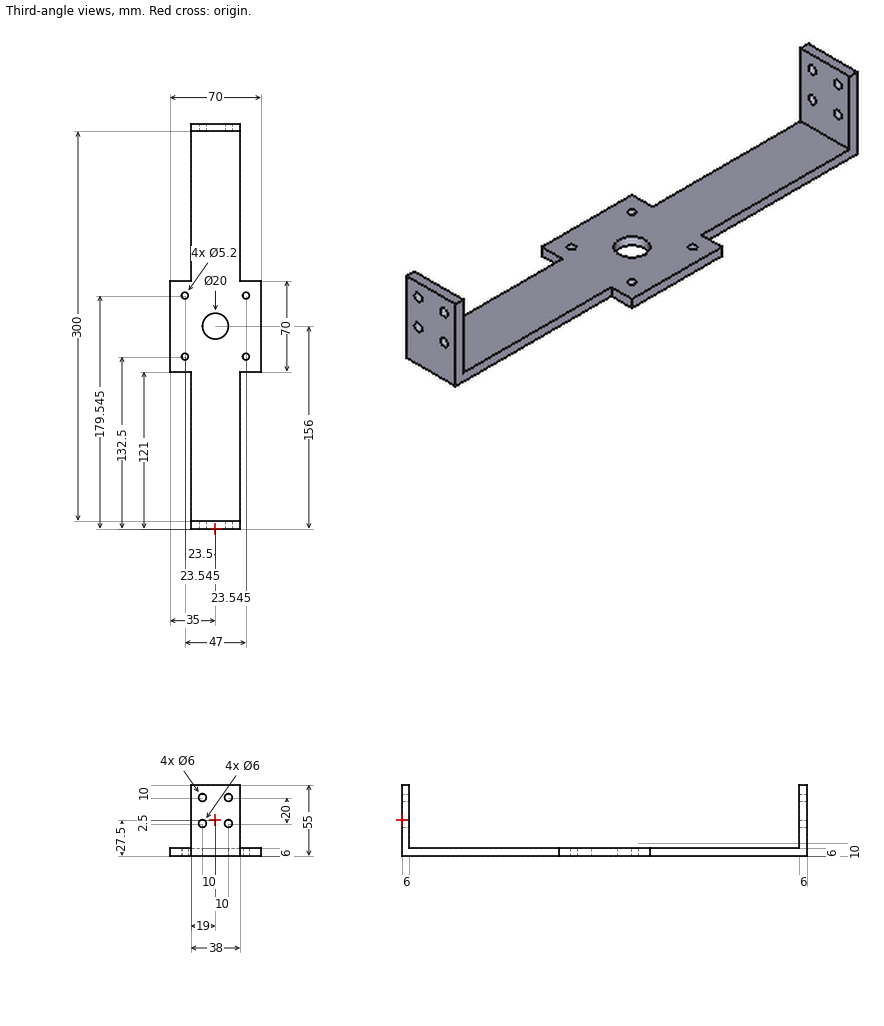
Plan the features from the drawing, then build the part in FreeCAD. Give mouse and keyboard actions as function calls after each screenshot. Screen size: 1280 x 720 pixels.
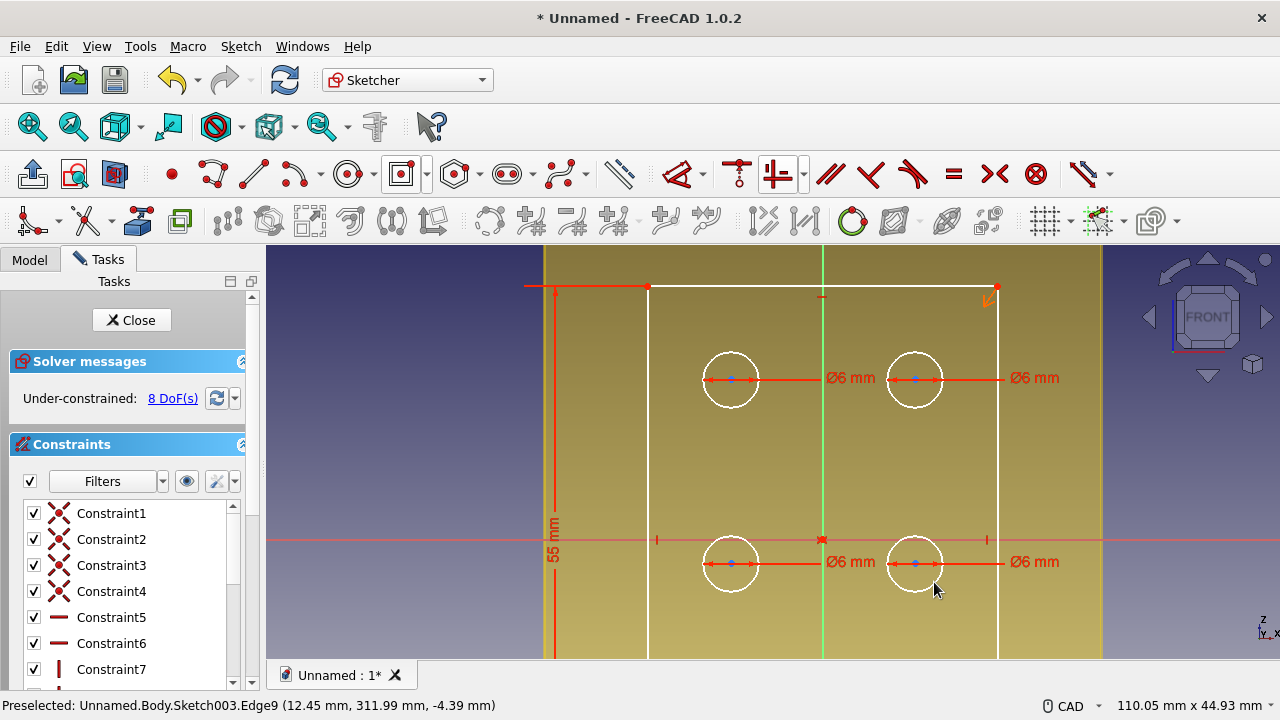
click(731, 380)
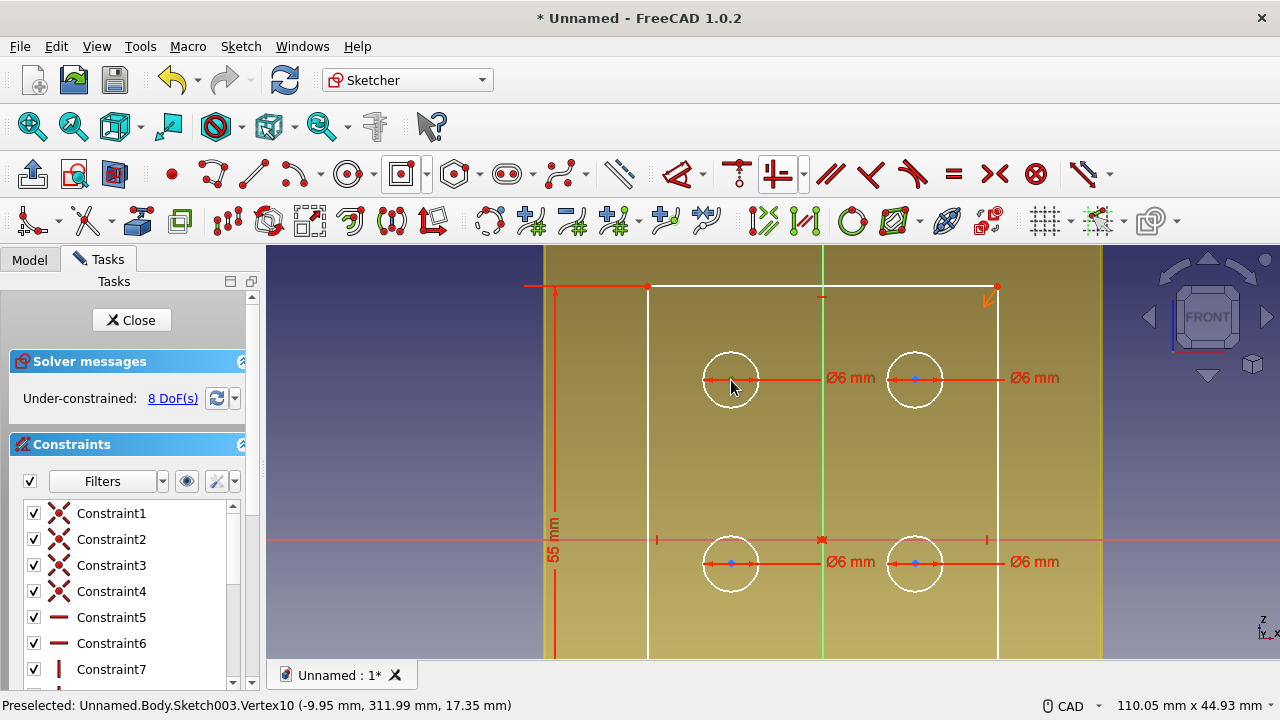
click(915, 380)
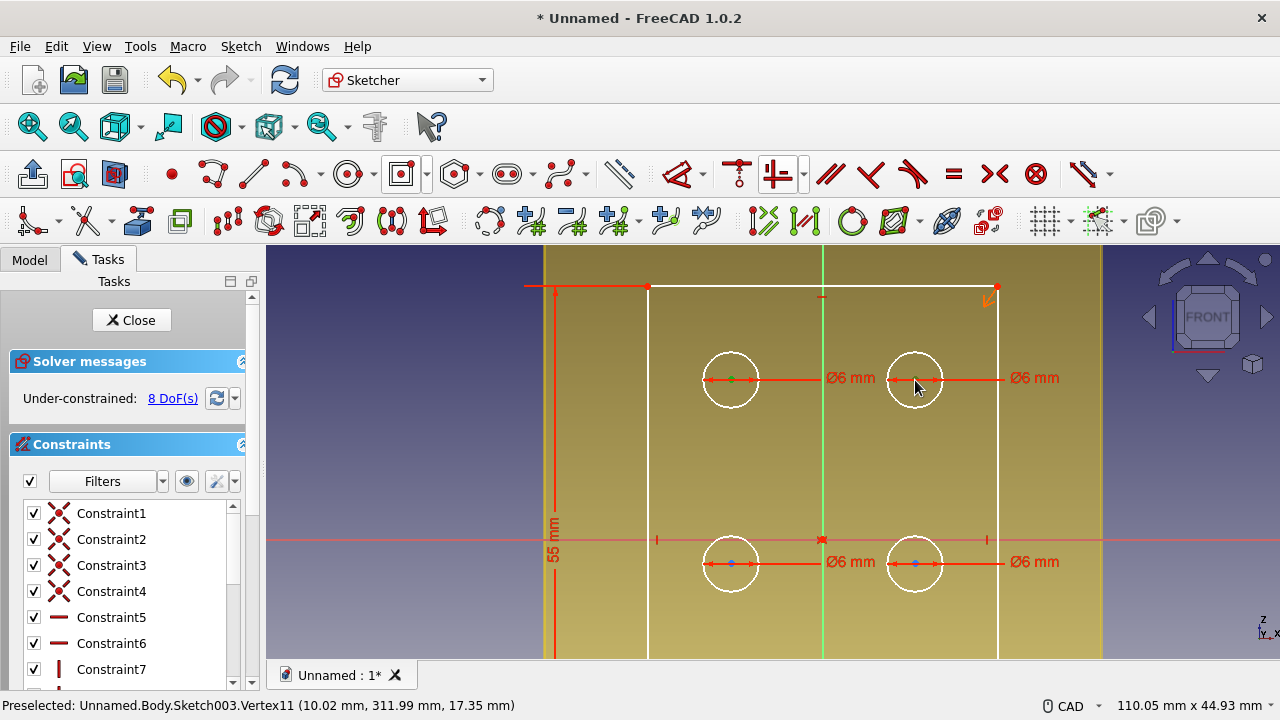
click(804, 174)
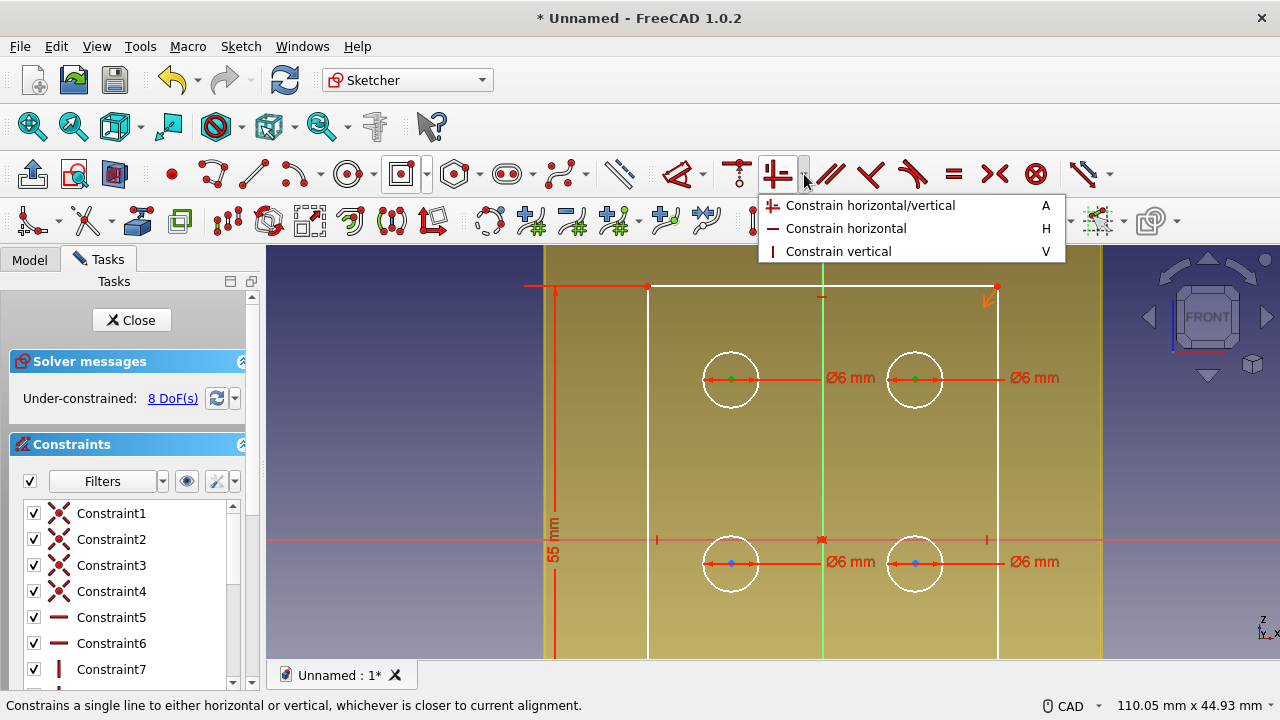
click(912, 228)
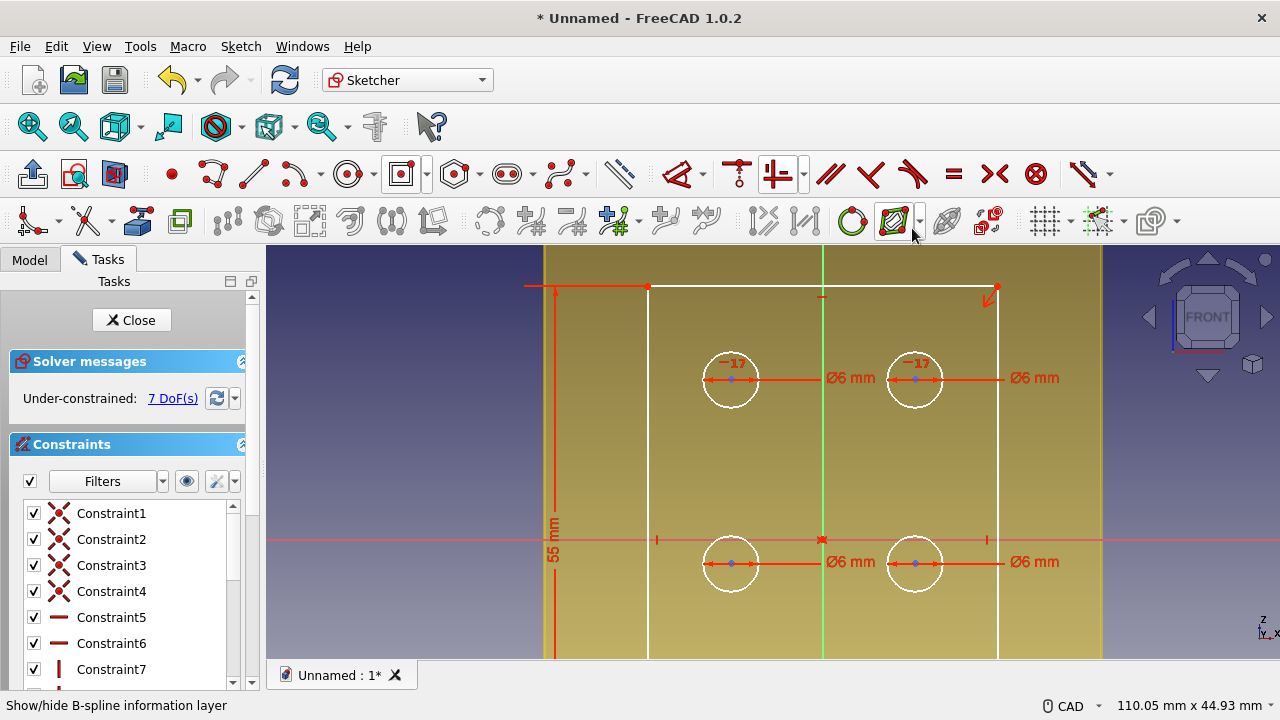
click(731, 380)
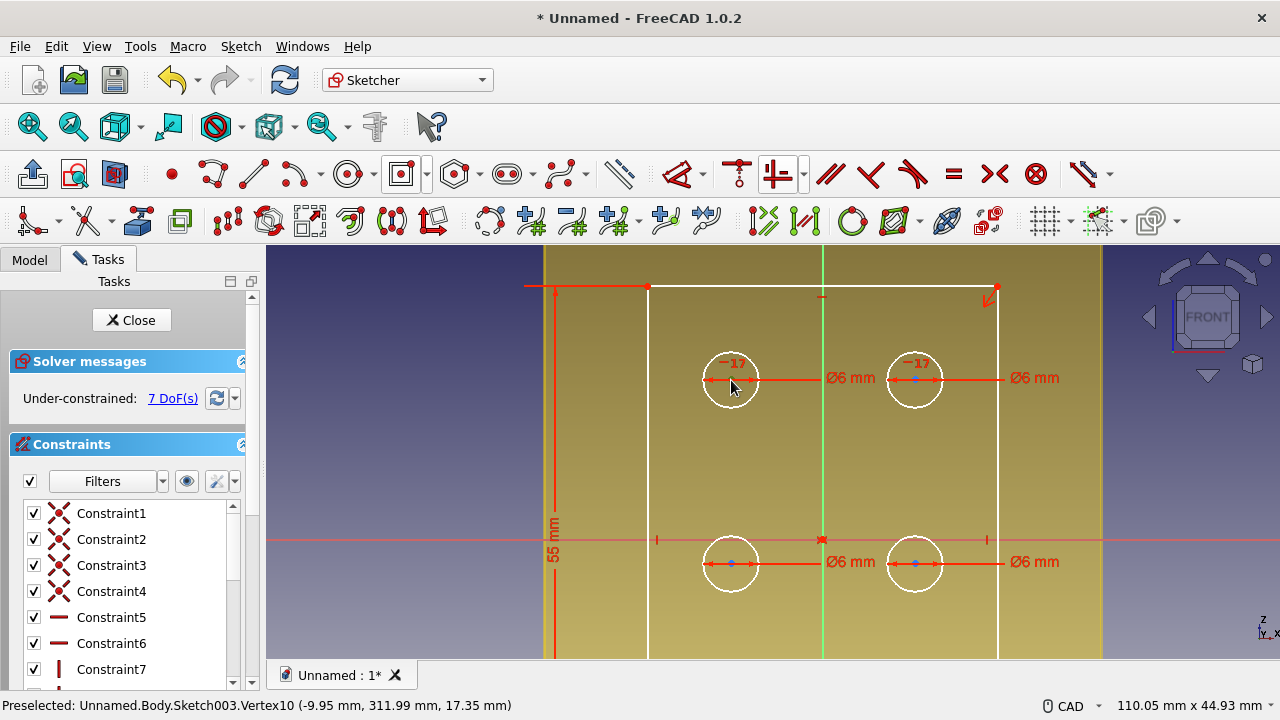
click(731, 564)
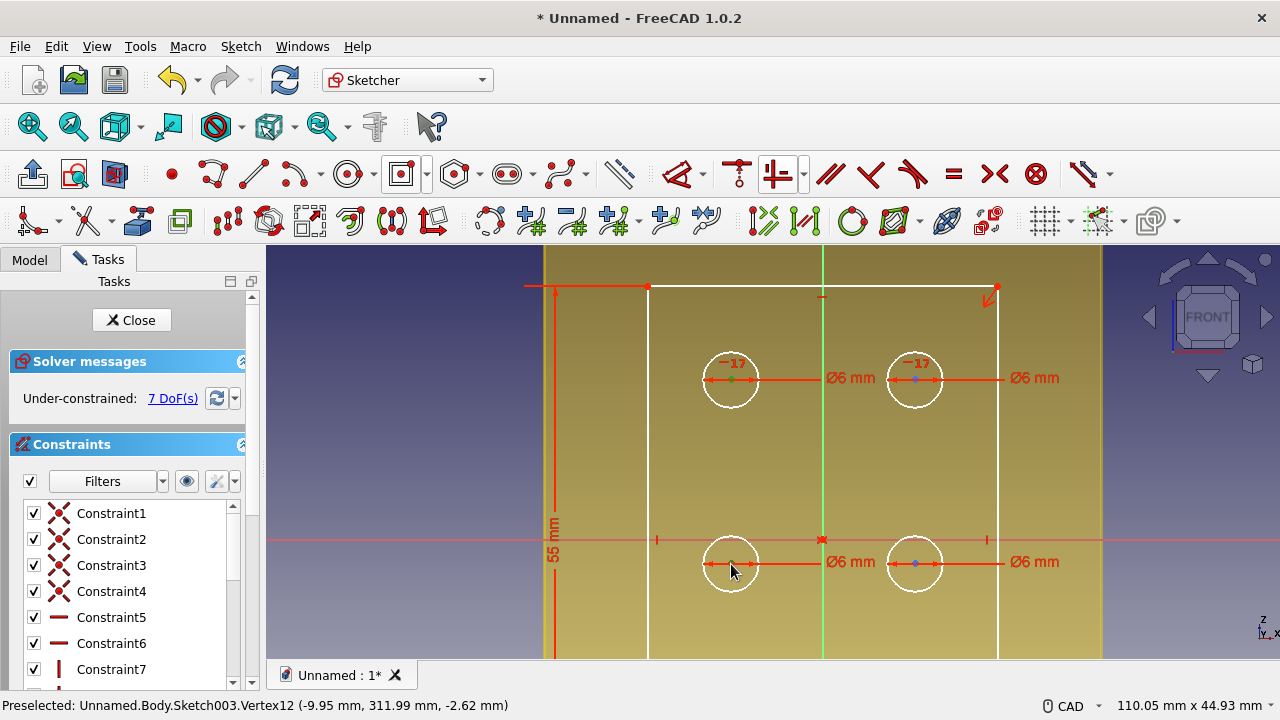
click(804, 174)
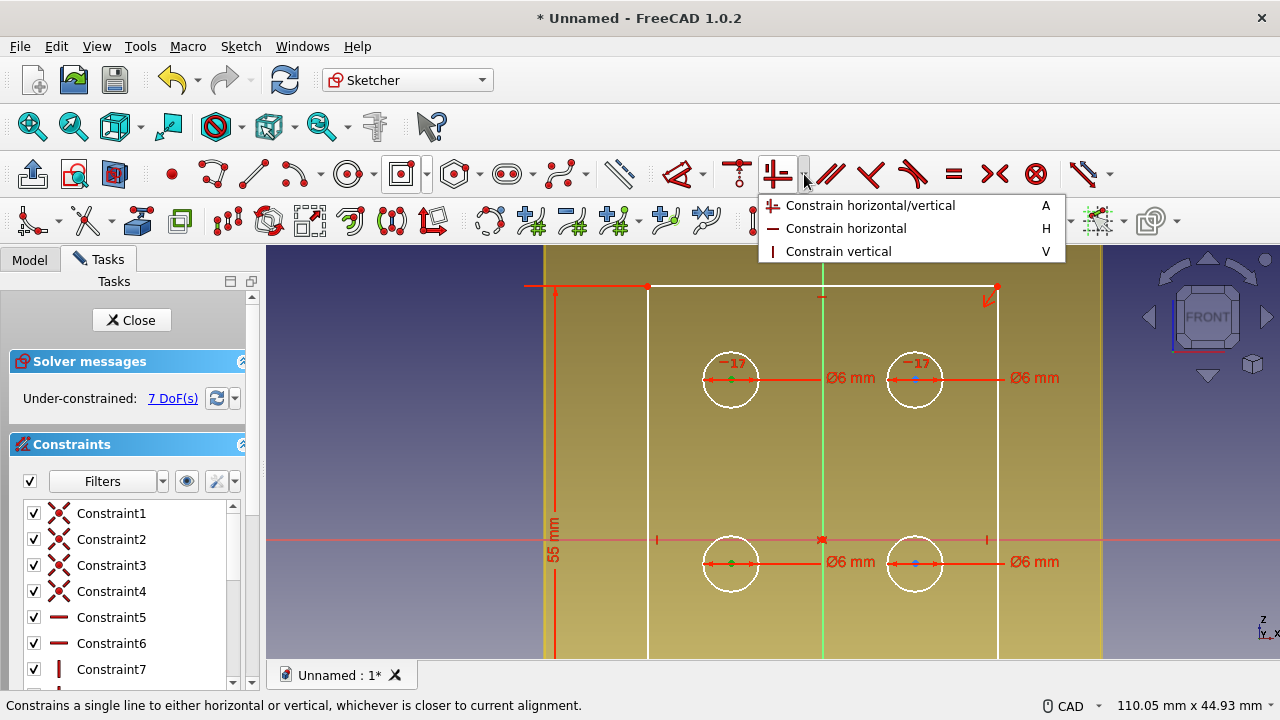
click(912, 252)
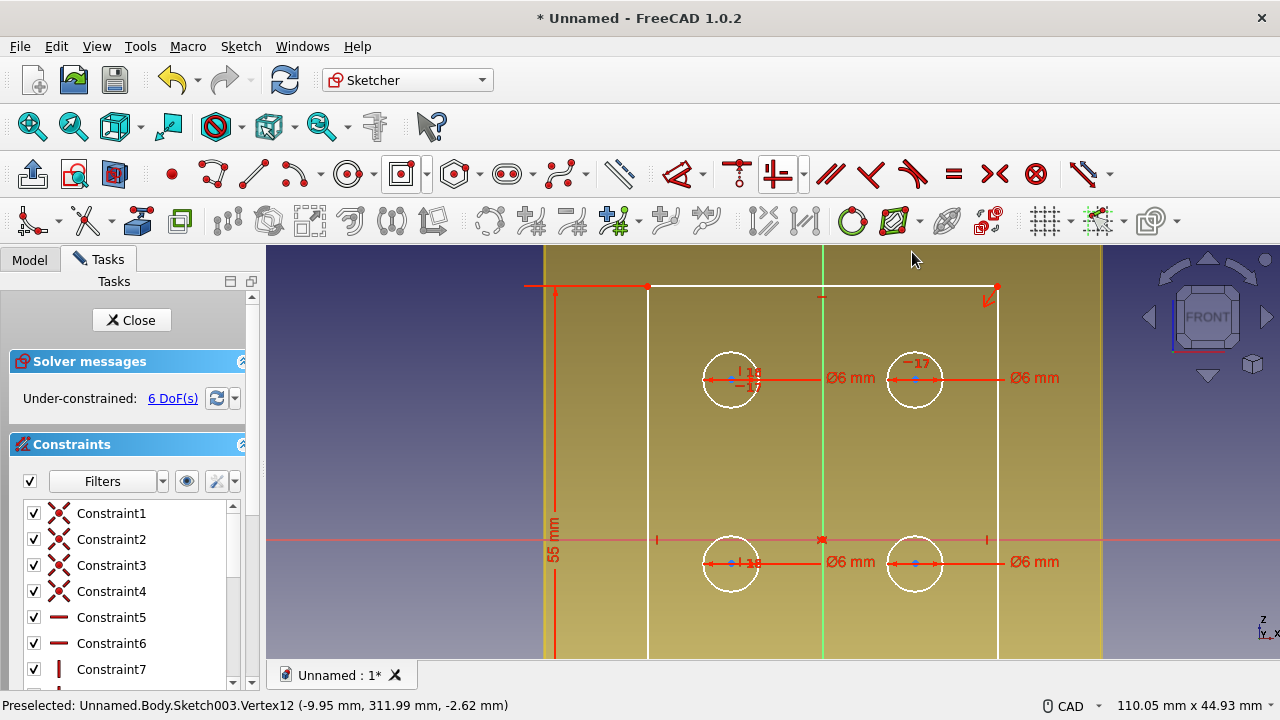
click(915, 380)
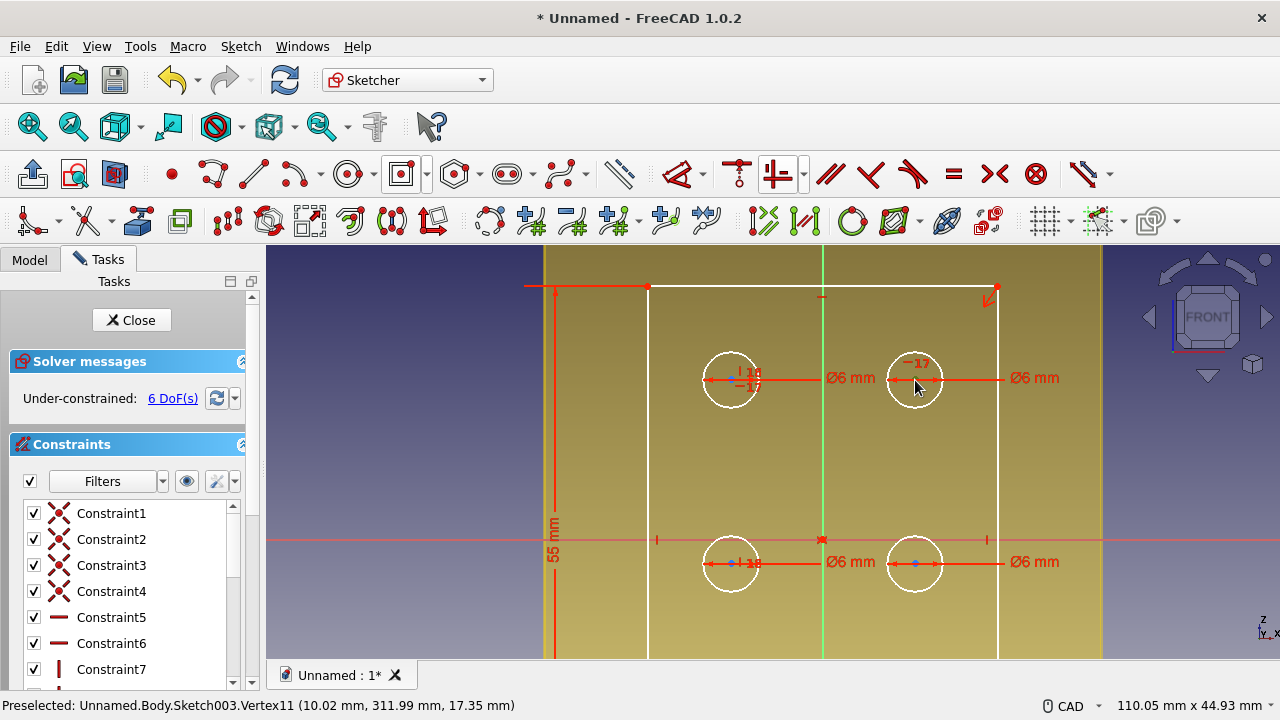
click(915, 564)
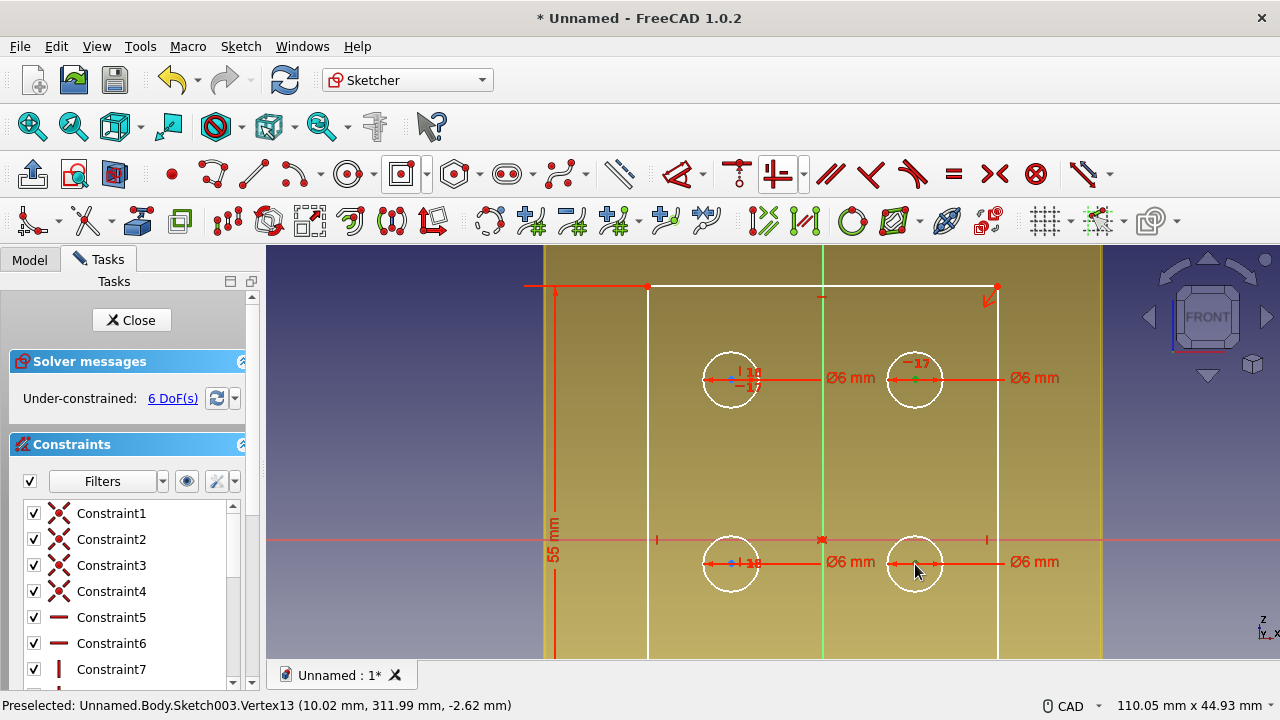
key(v)